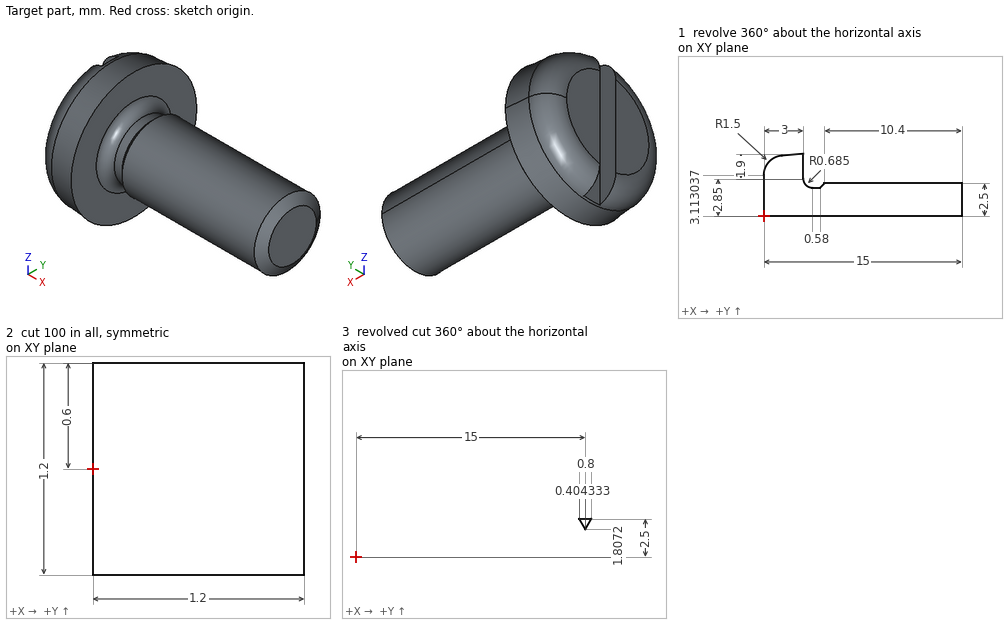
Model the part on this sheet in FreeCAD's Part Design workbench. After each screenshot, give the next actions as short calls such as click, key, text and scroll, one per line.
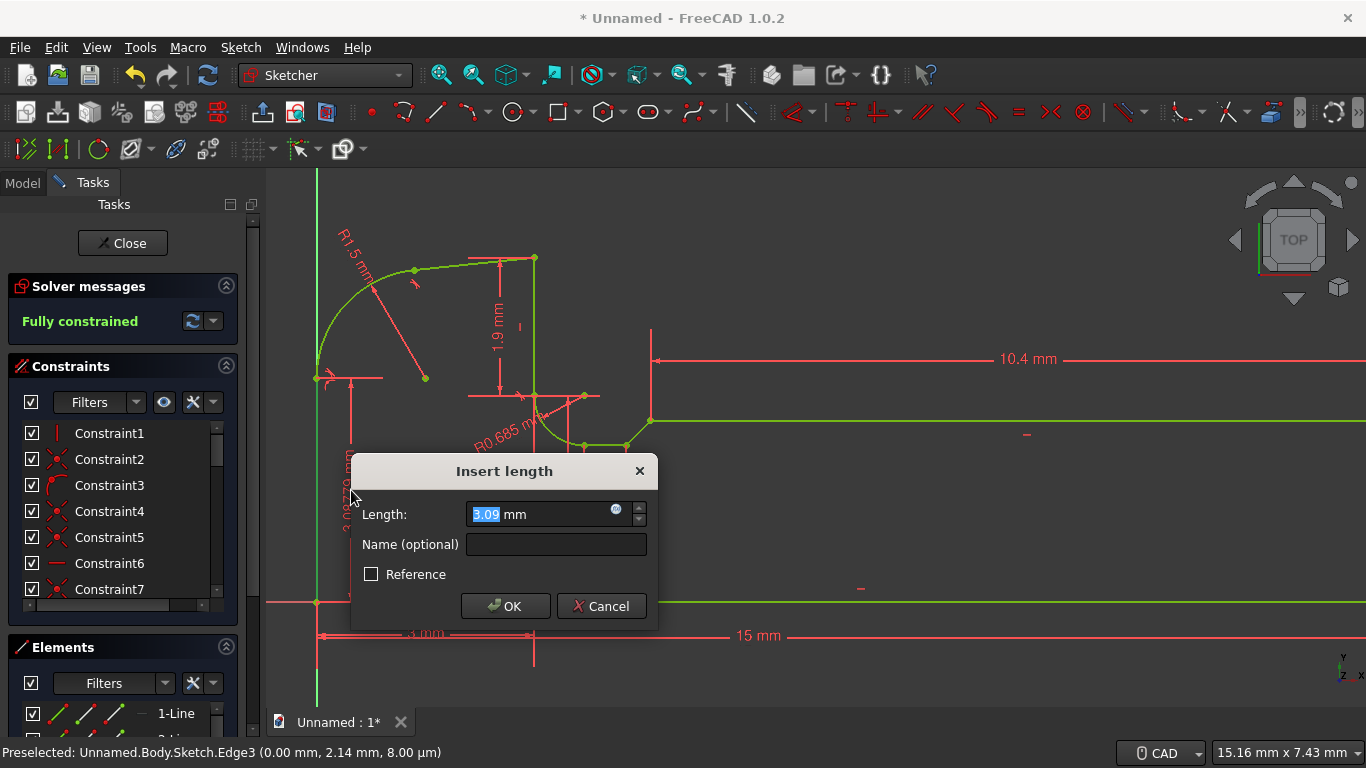
text(3.113037)
key(Return)
key(Escape)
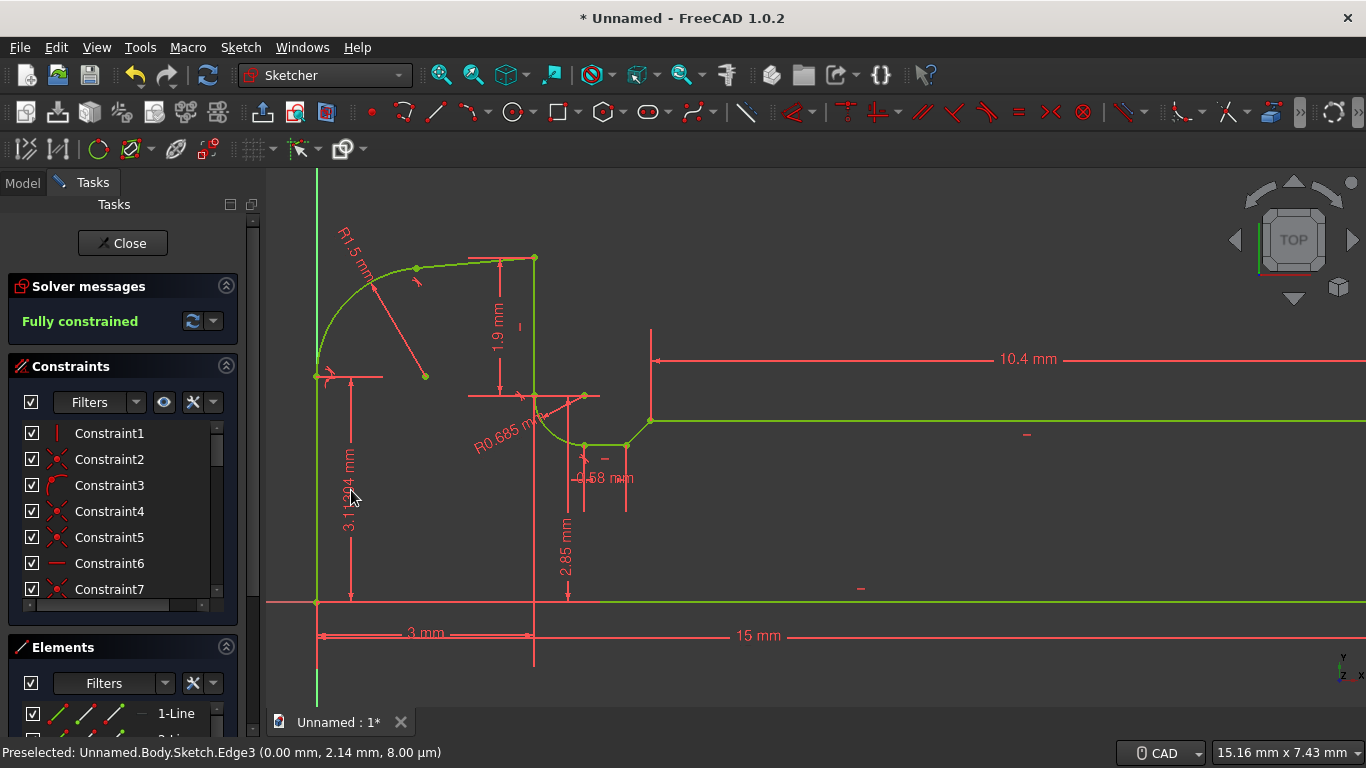
click(123, 243)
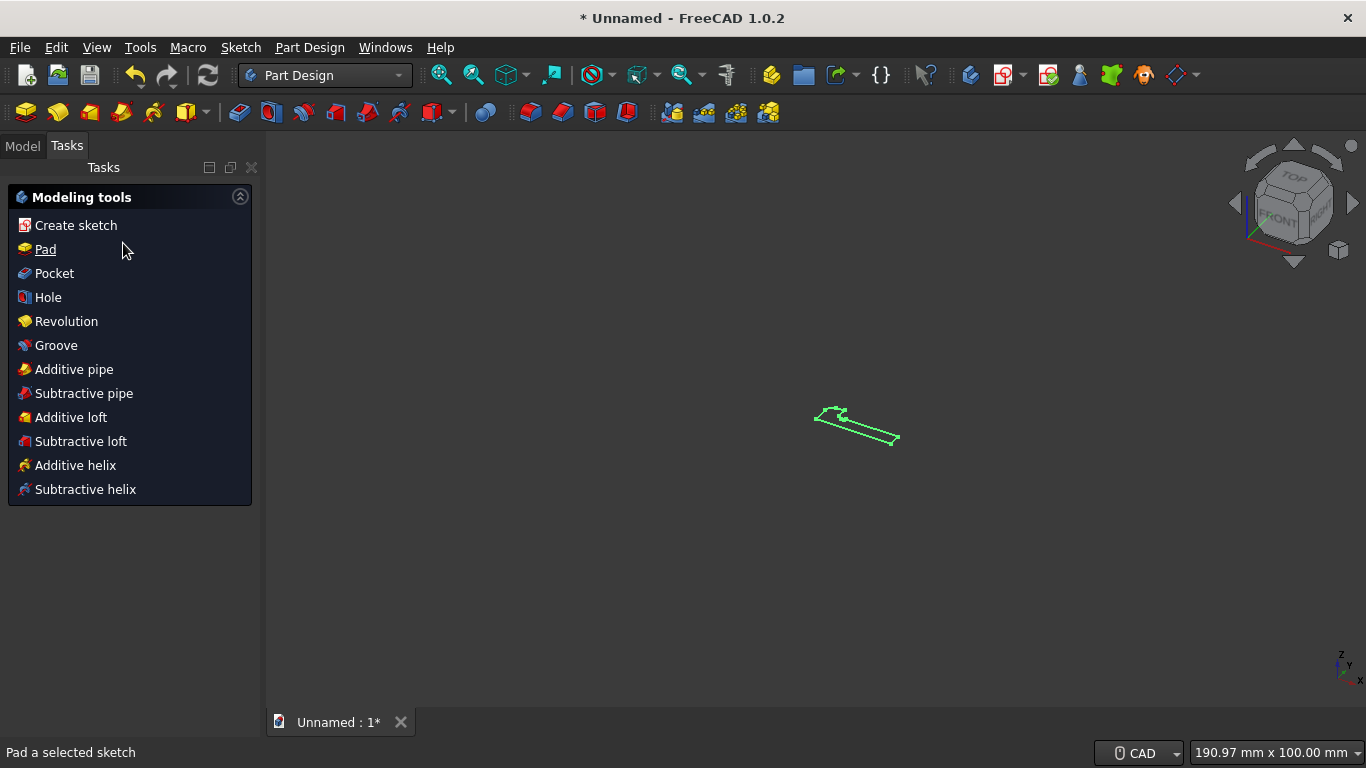
click(58, 112)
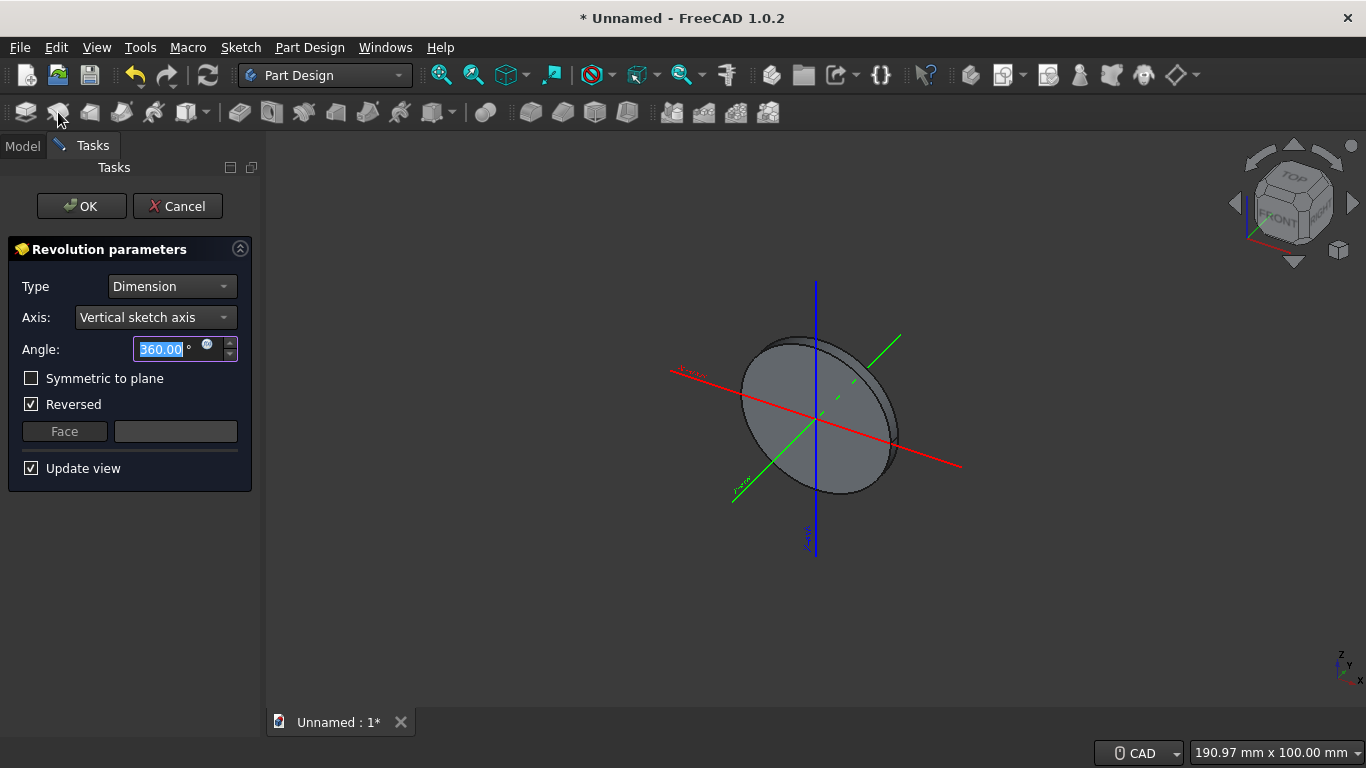
click(156, 318)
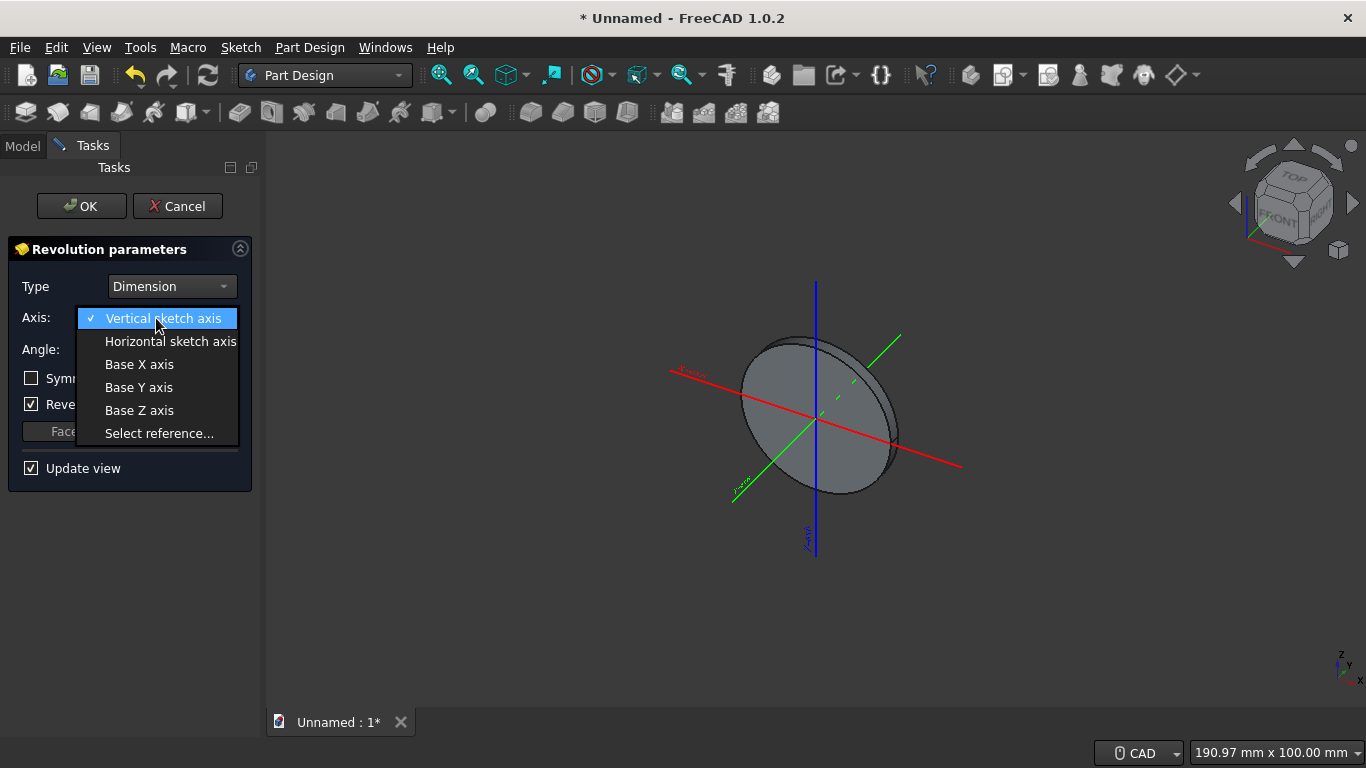
click(156, 342)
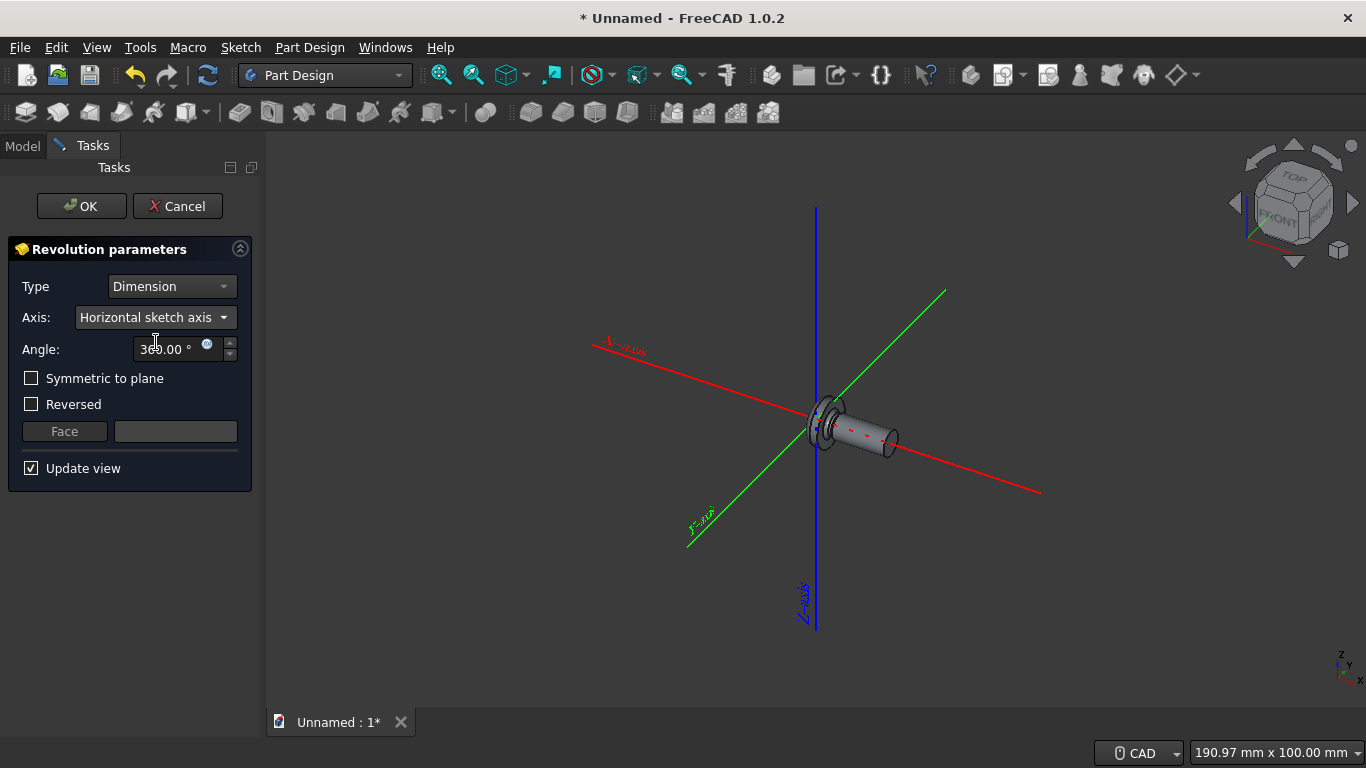
click(82, 206)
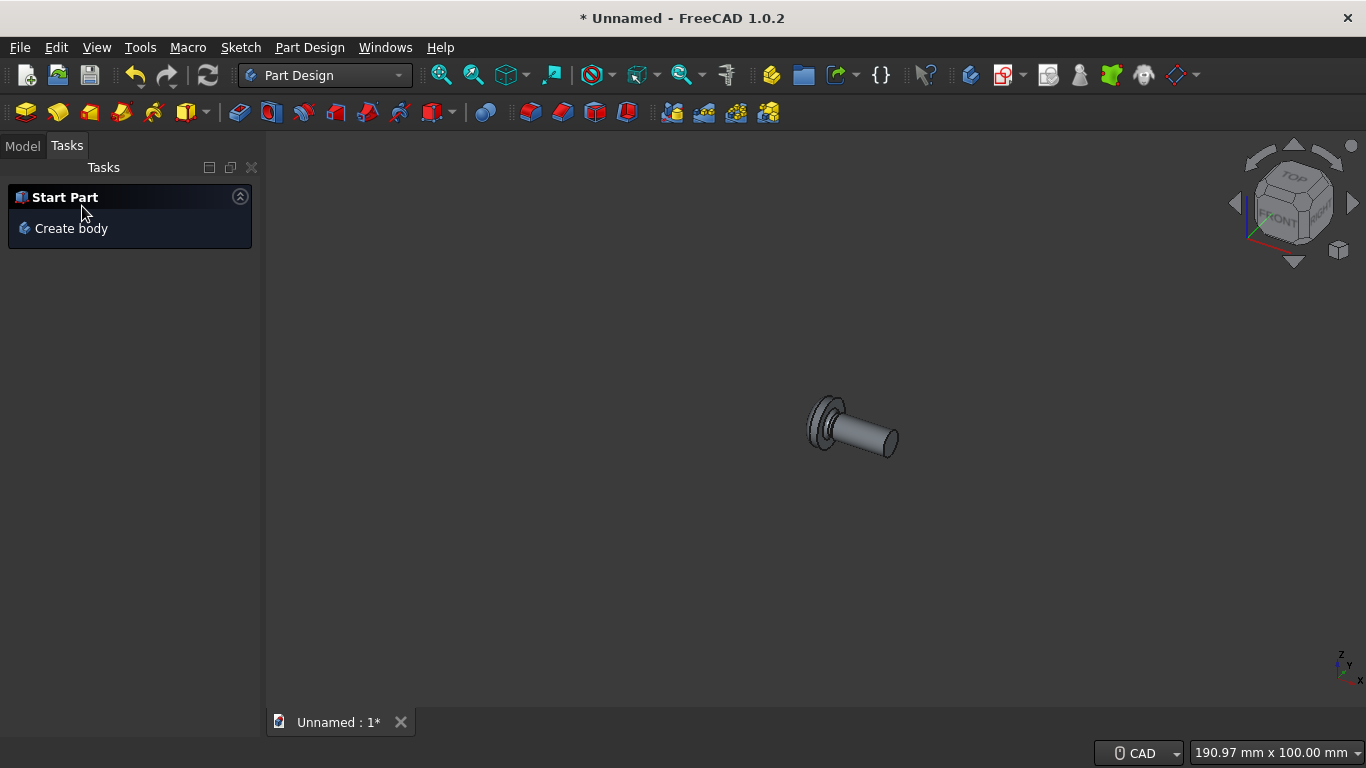
key(v)
key(f)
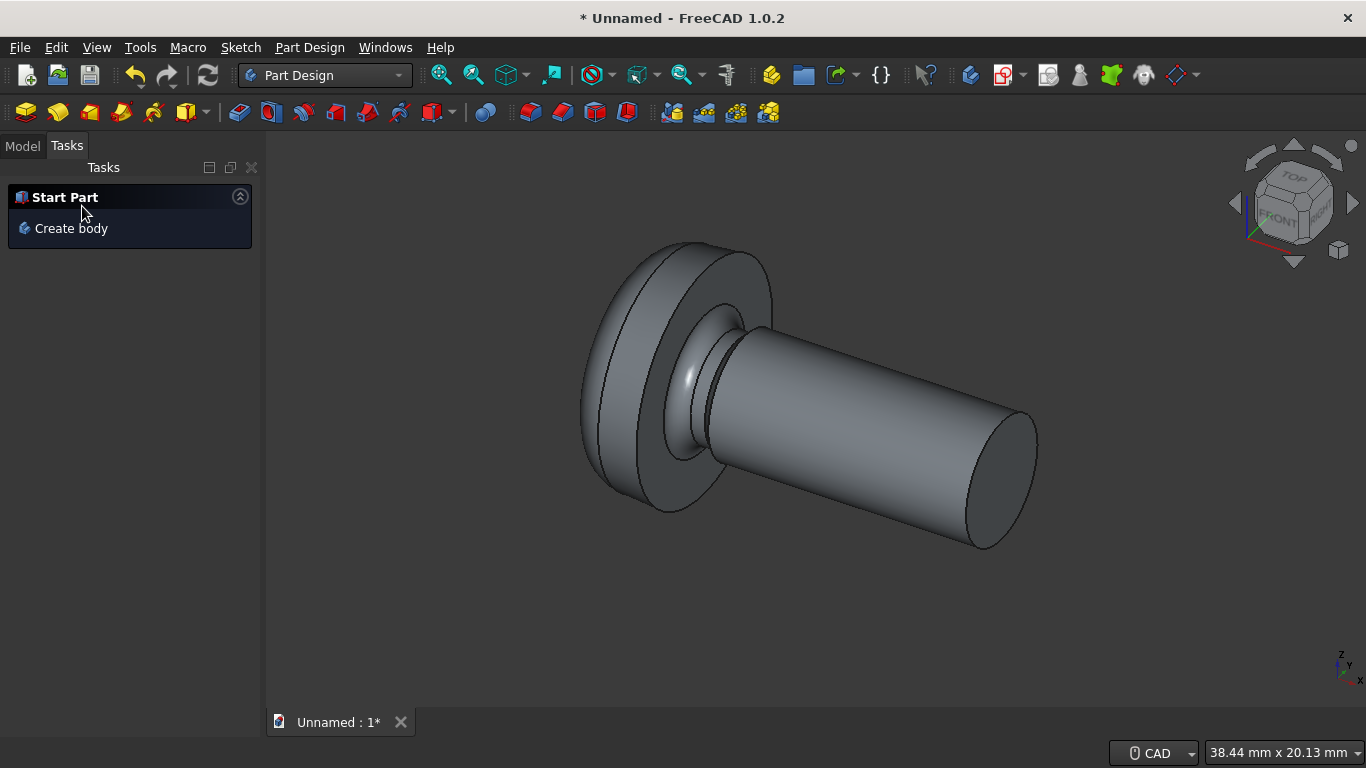
click(1004, 76)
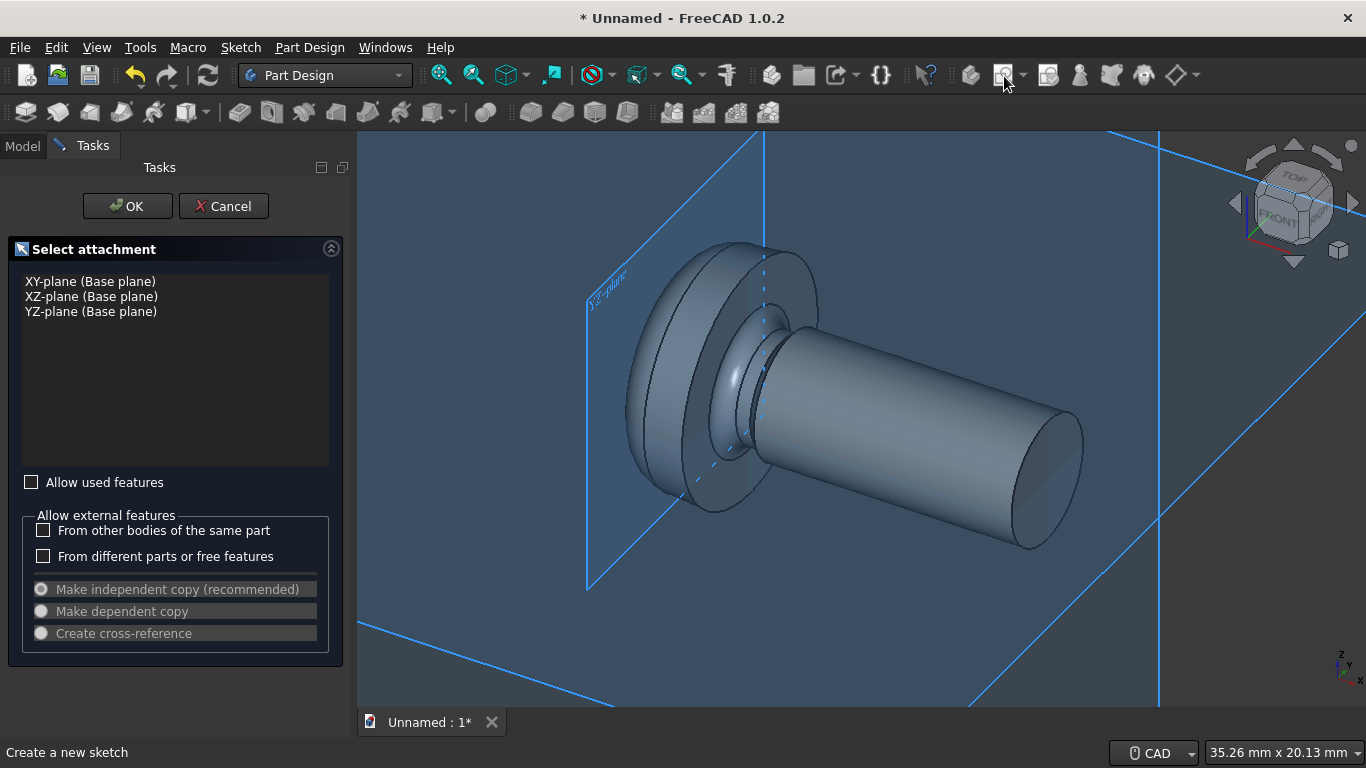
click(82, 282)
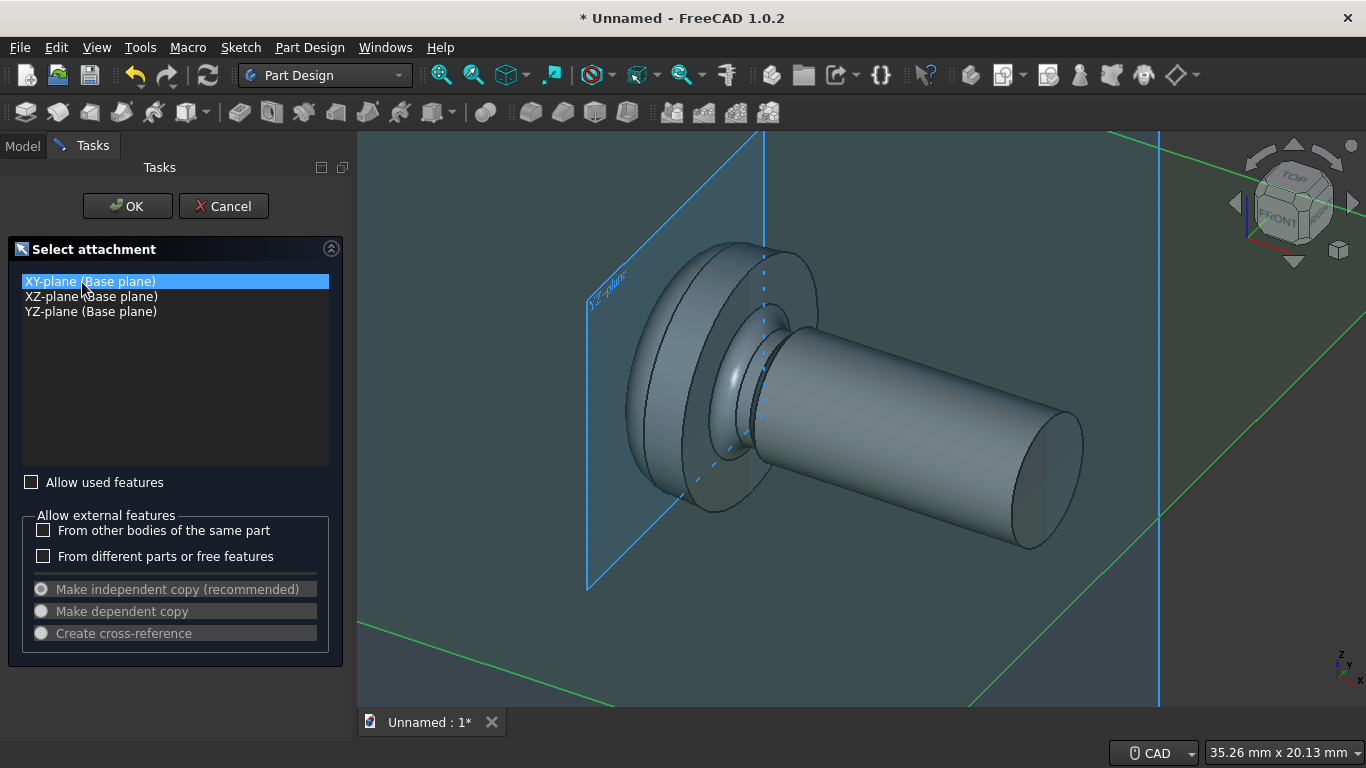
click(128, 206)